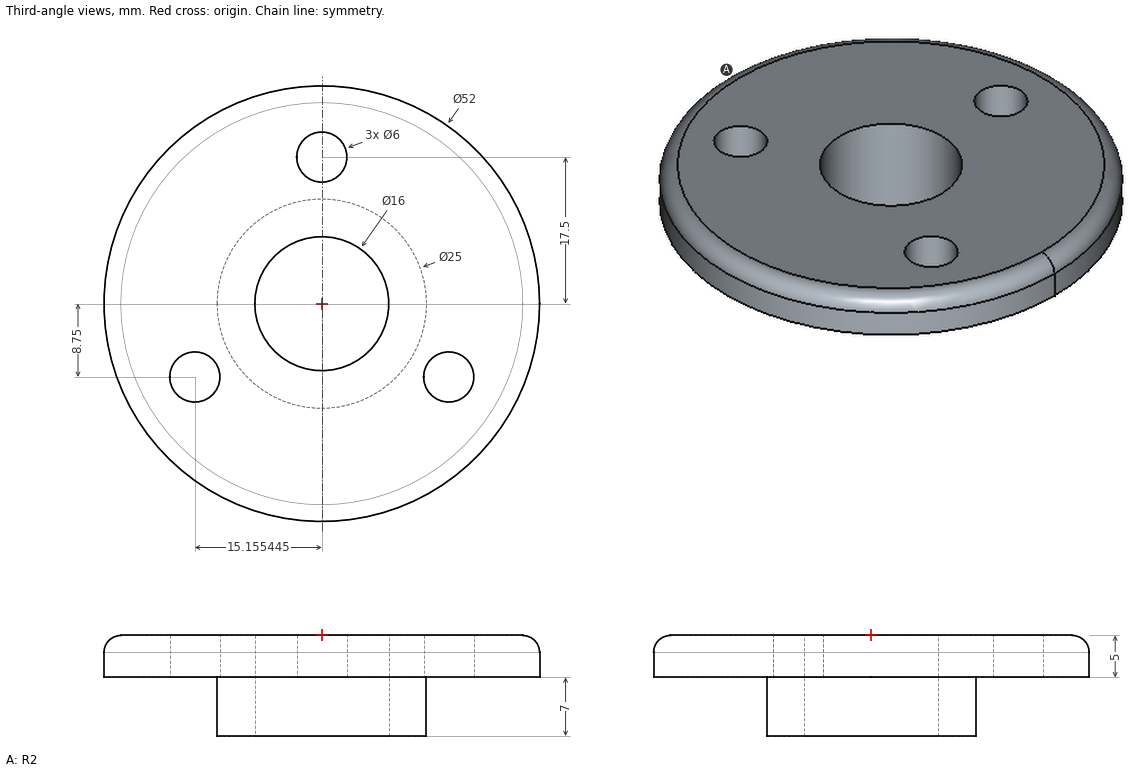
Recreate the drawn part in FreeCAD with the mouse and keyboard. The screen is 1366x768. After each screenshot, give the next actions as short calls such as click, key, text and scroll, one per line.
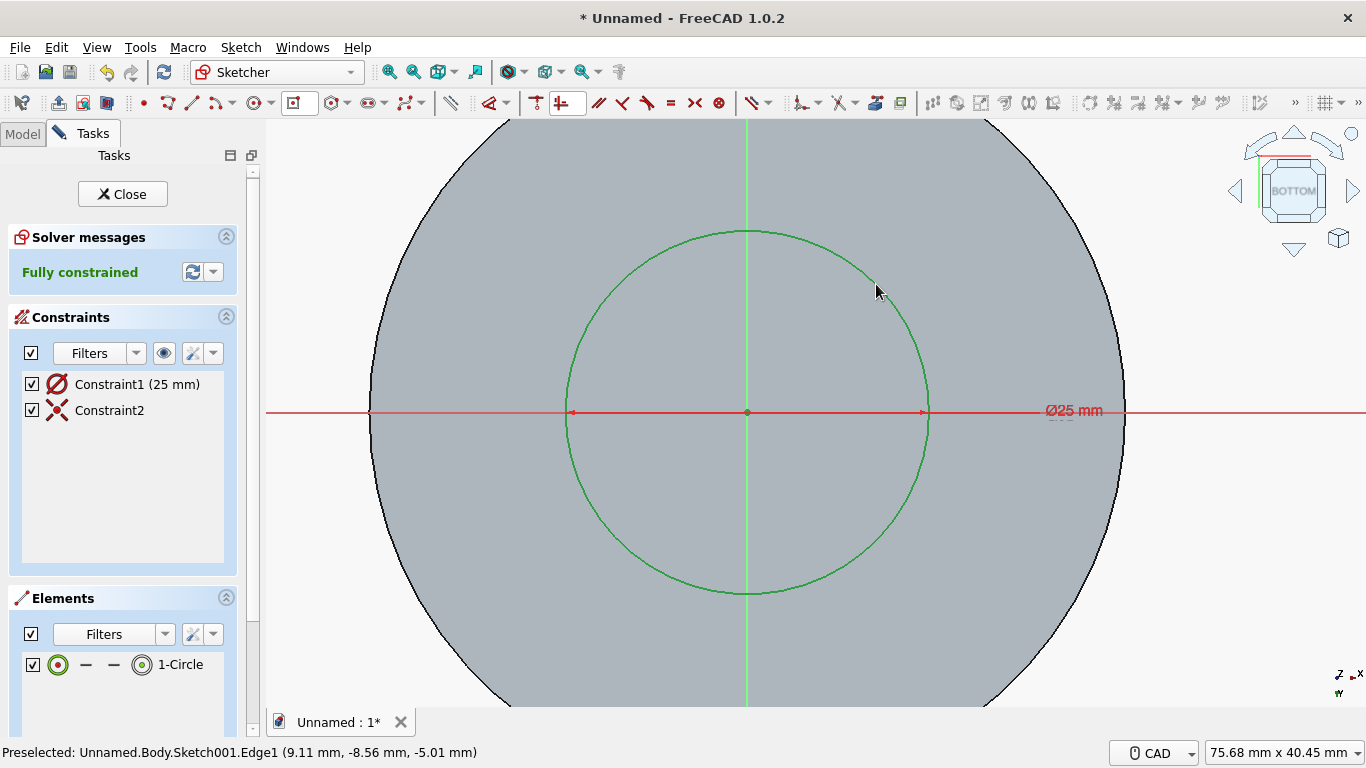
click(123, 194)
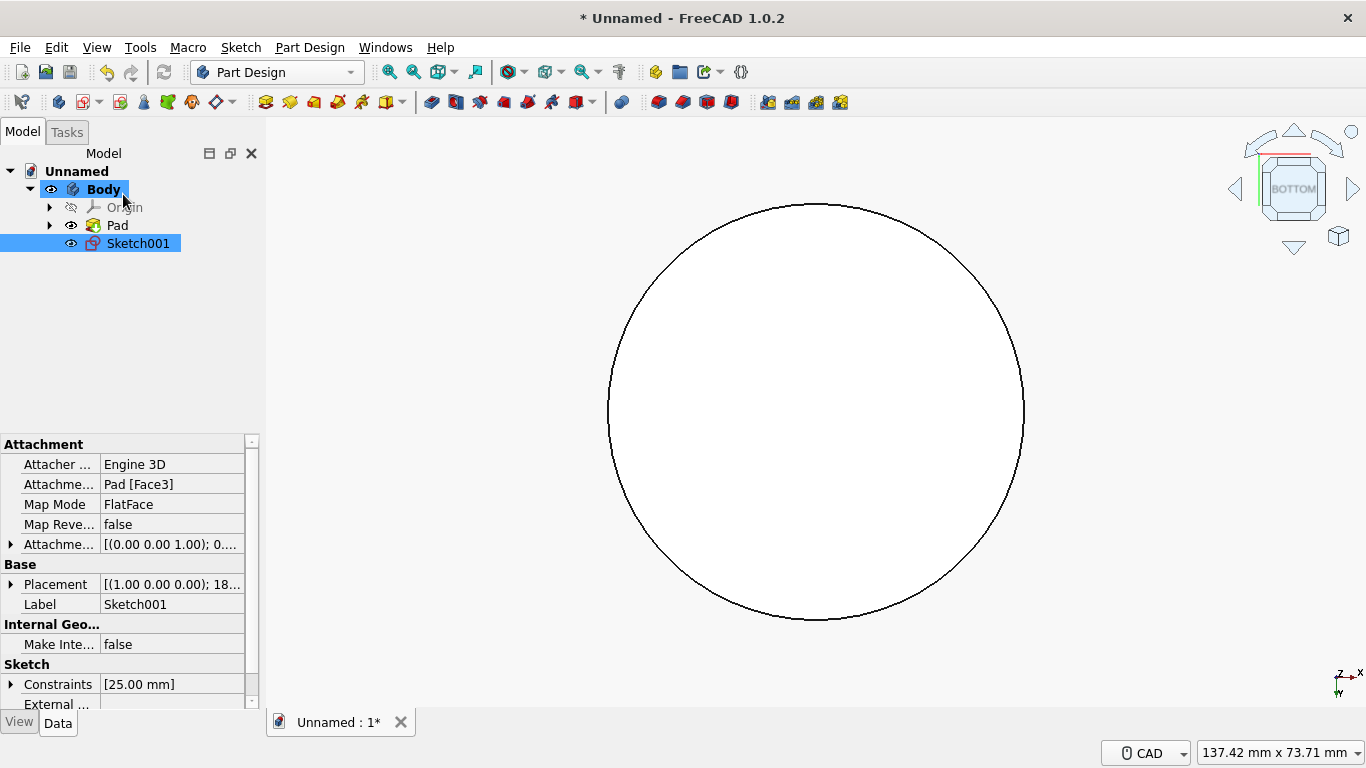
click(266, 102)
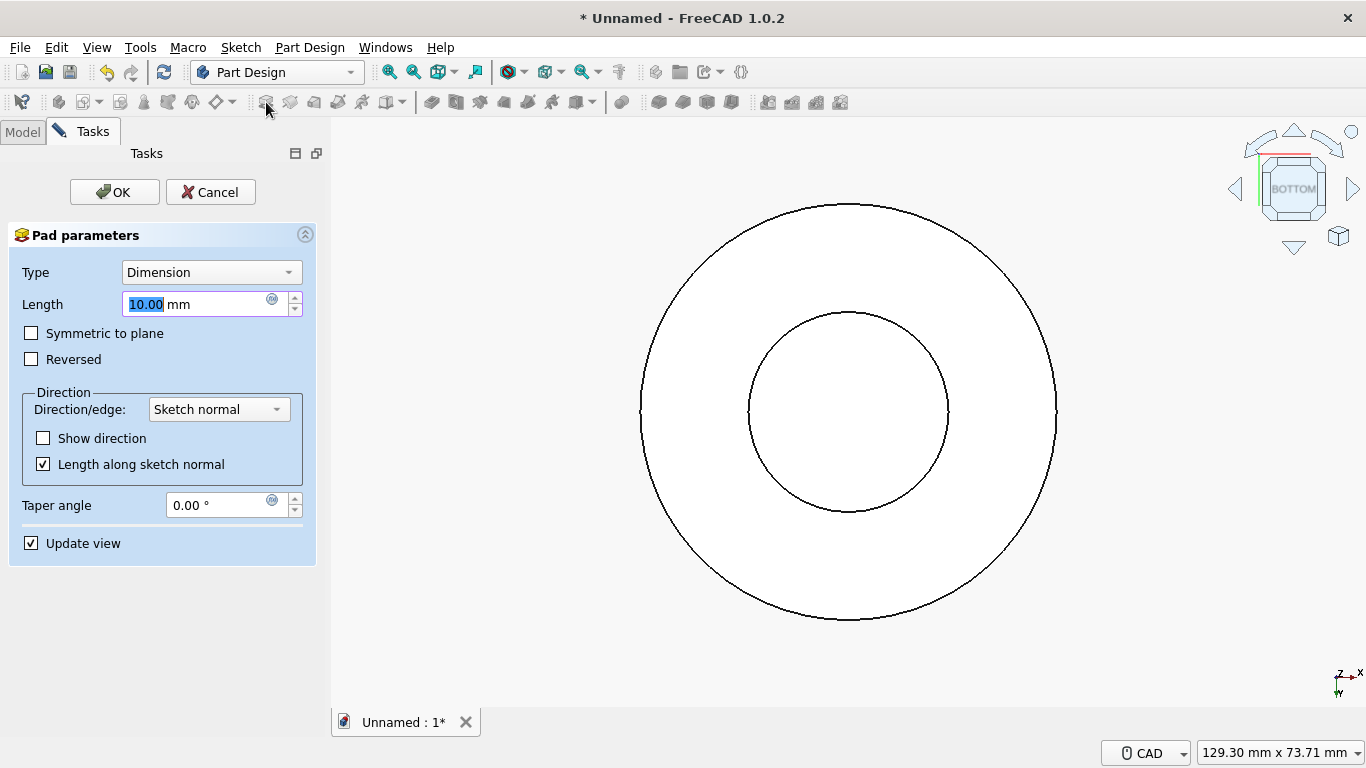
text(7)
key(Tab)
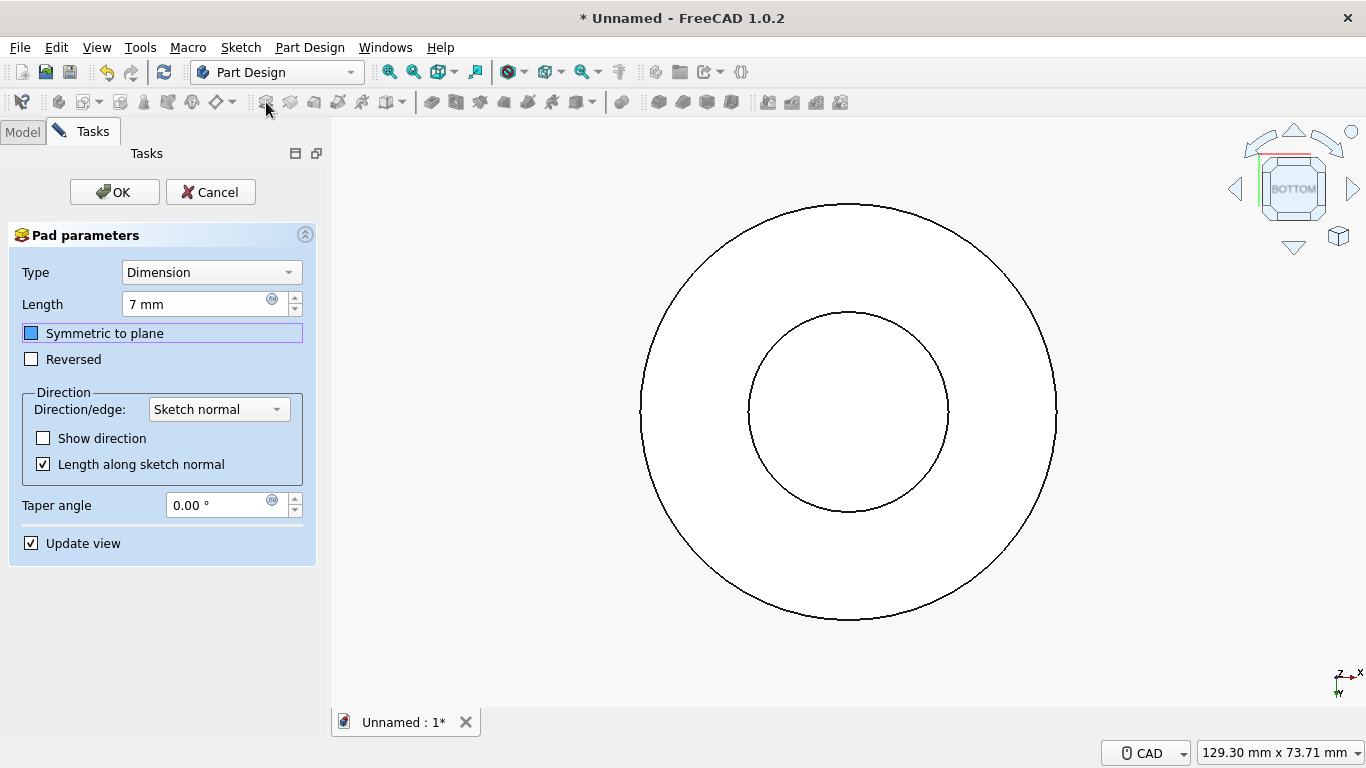
click(115, 192)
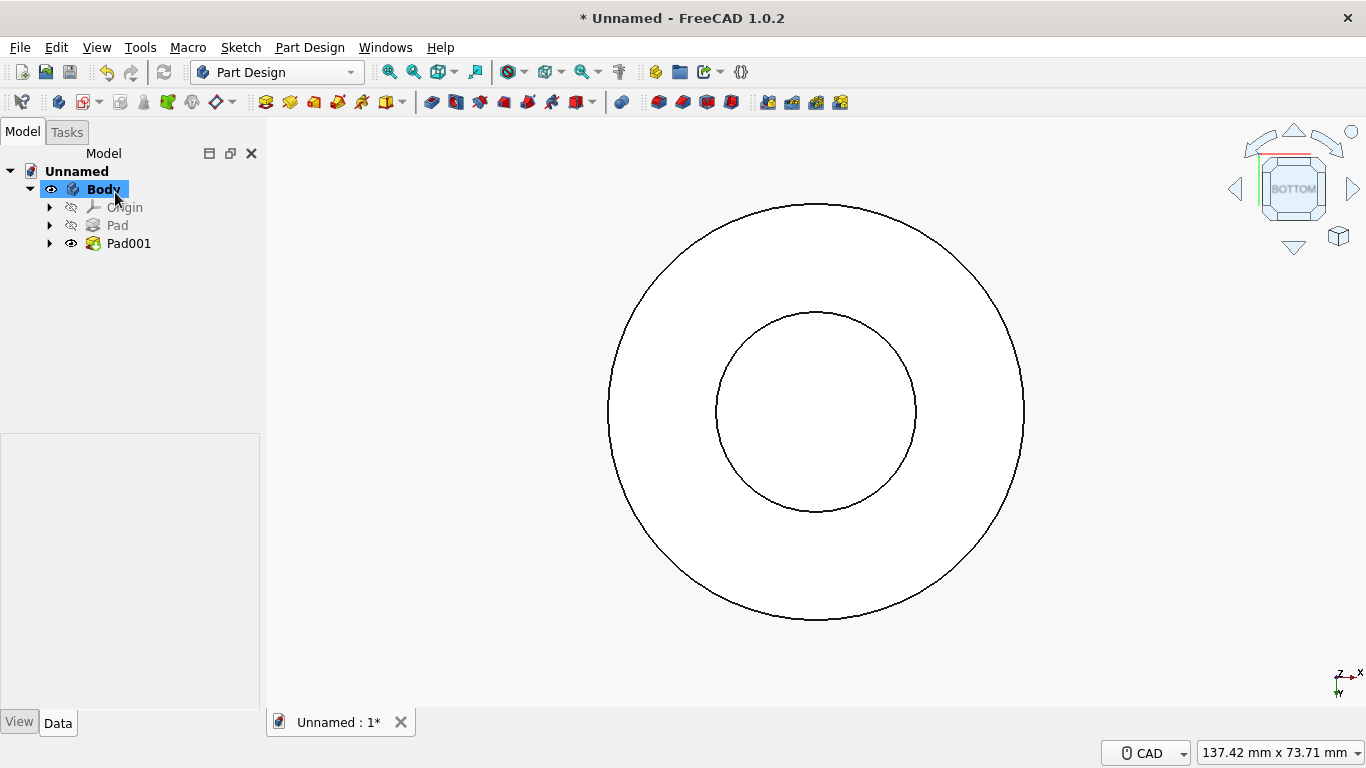
click(816, 411)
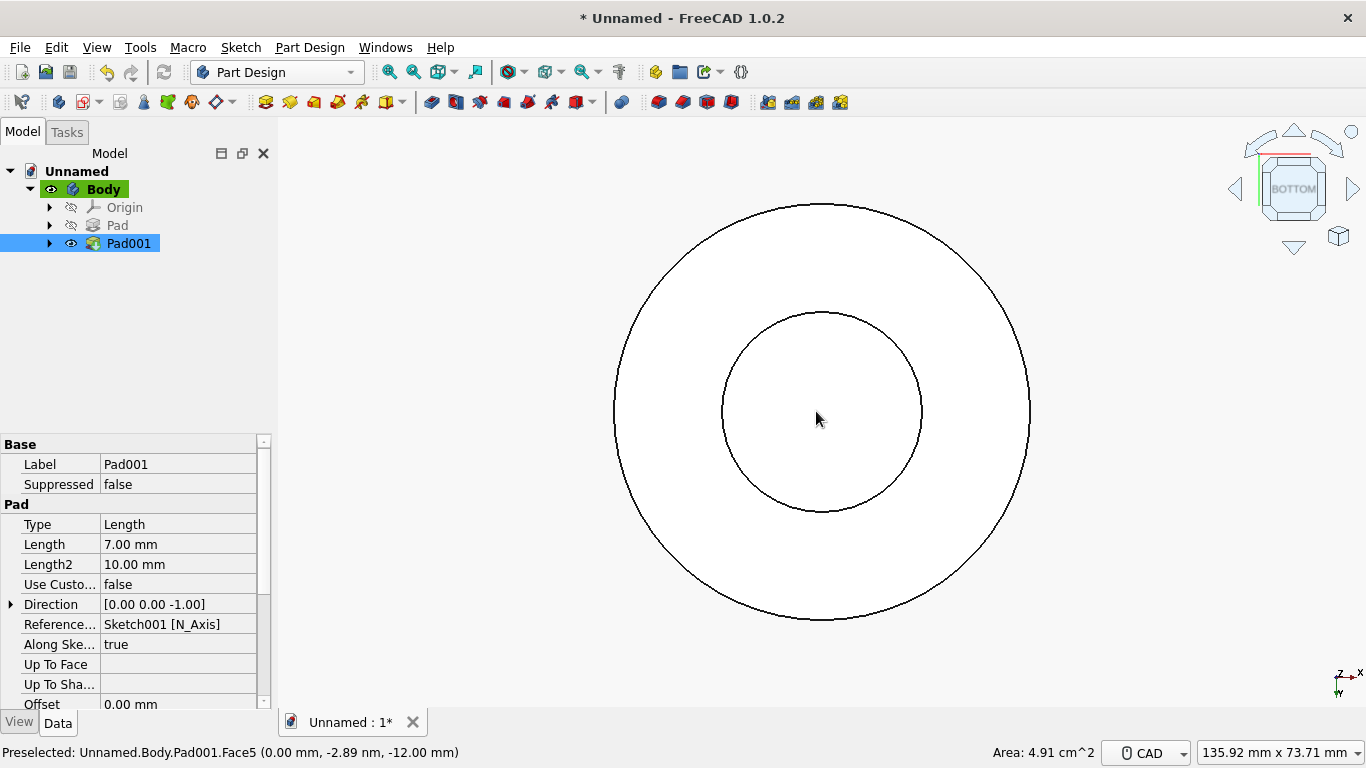
click(84, 102)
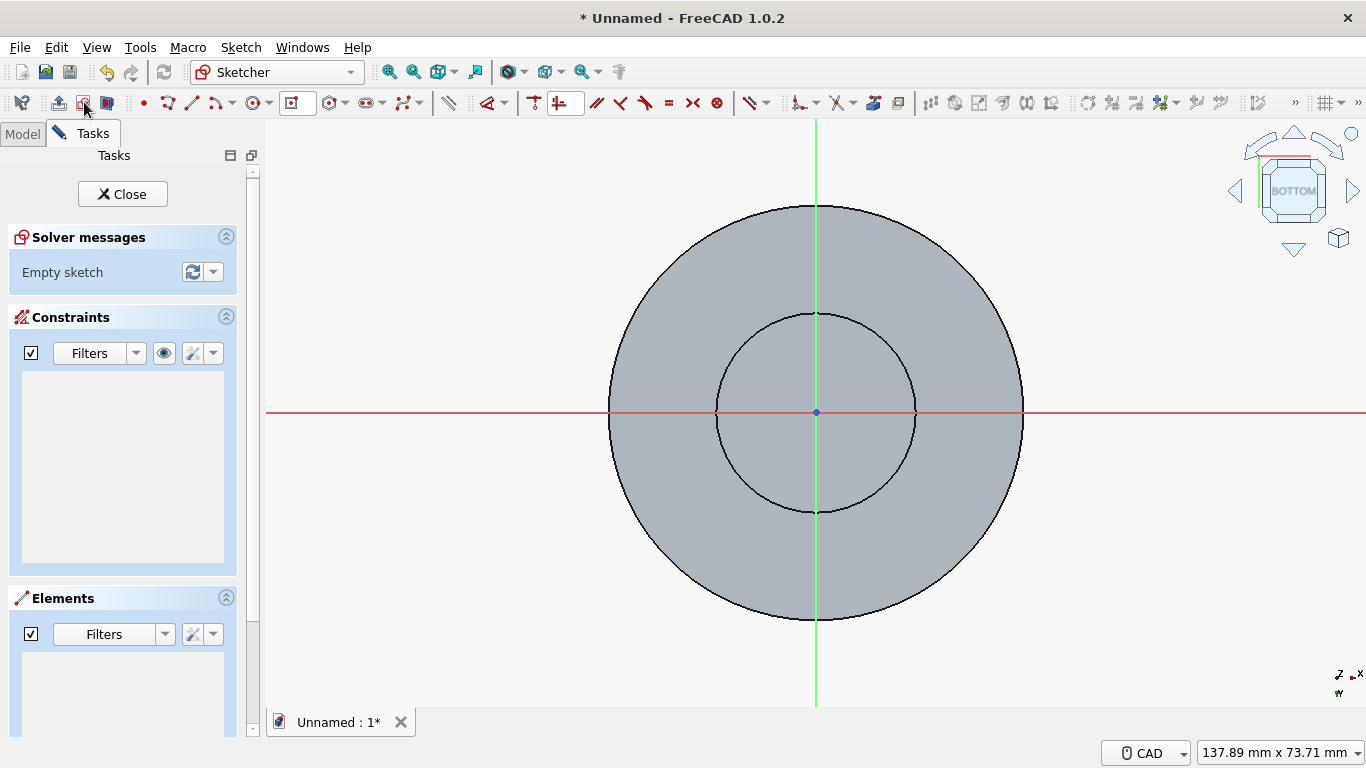
scroll(856, 413, up, 5)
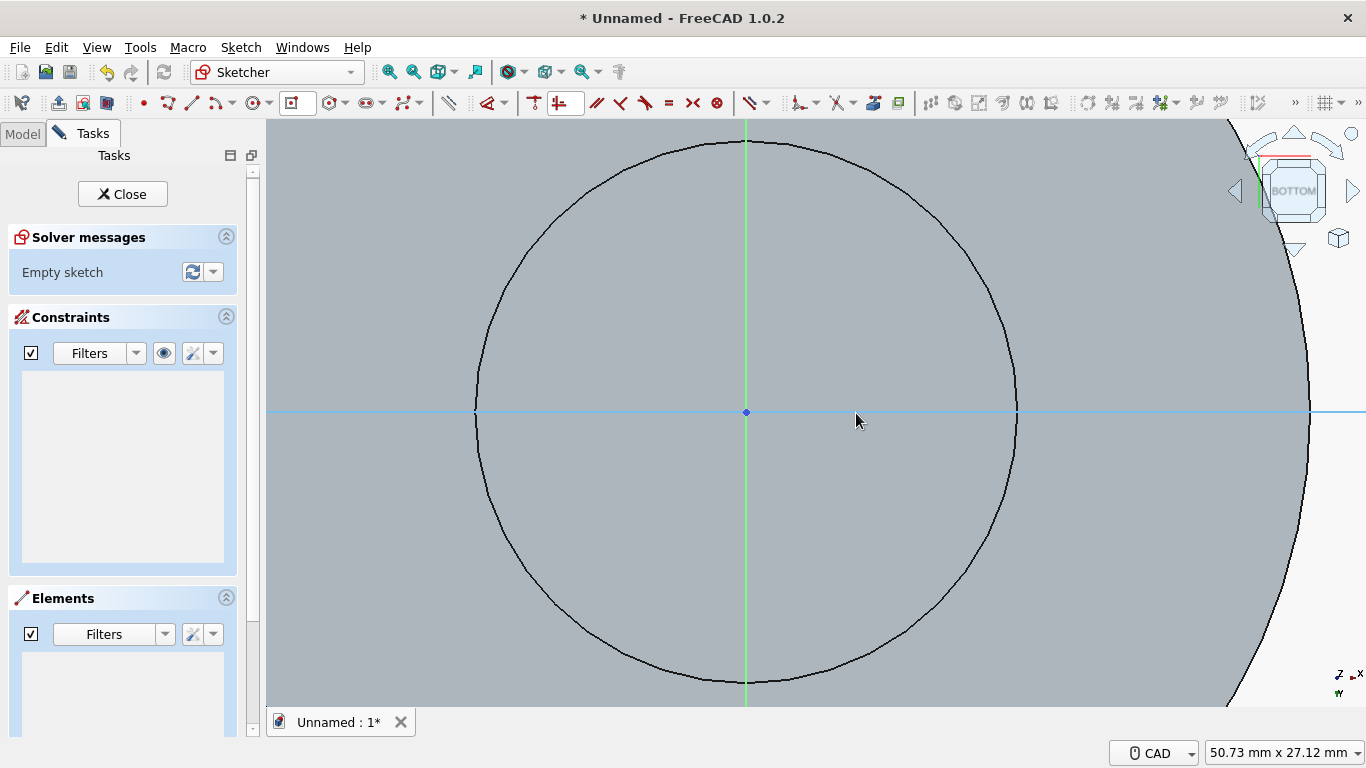
click(254, 104)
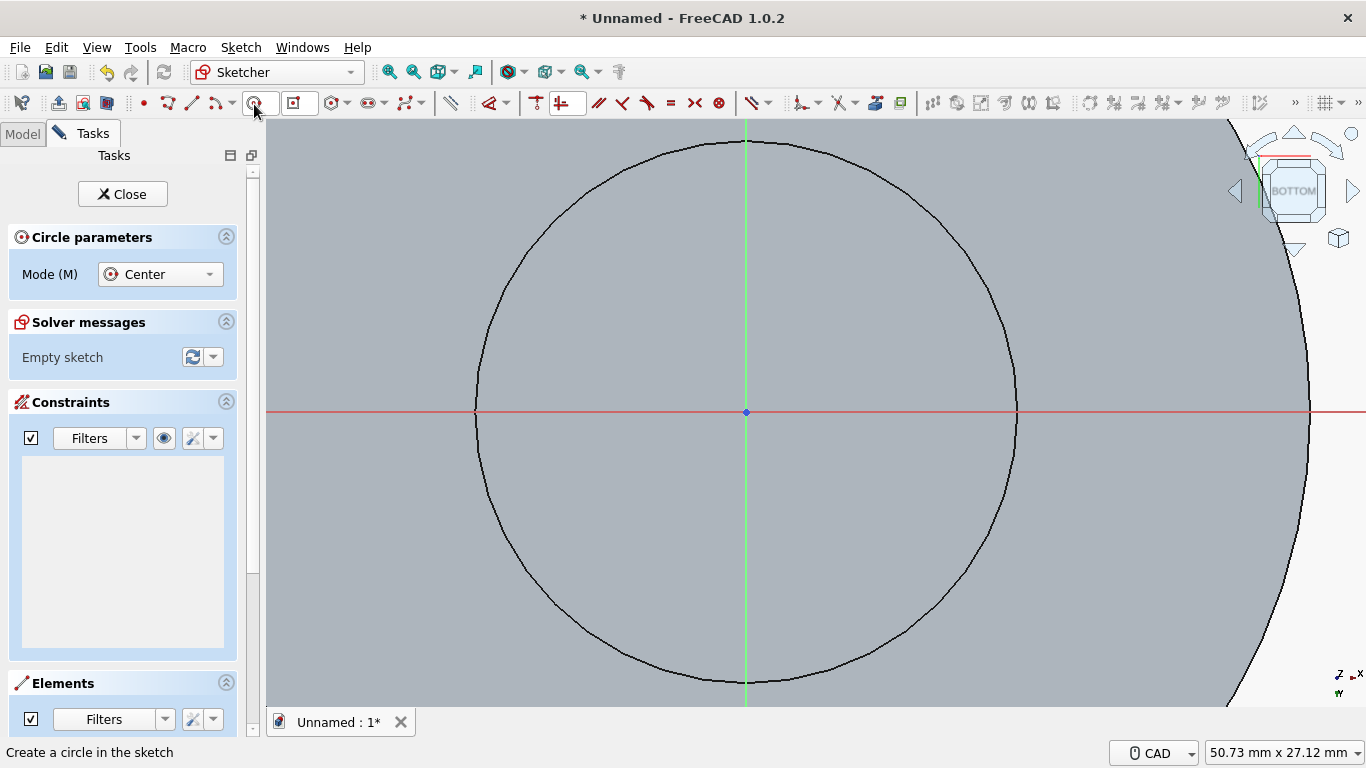
click(746, 412)
move(869, 289)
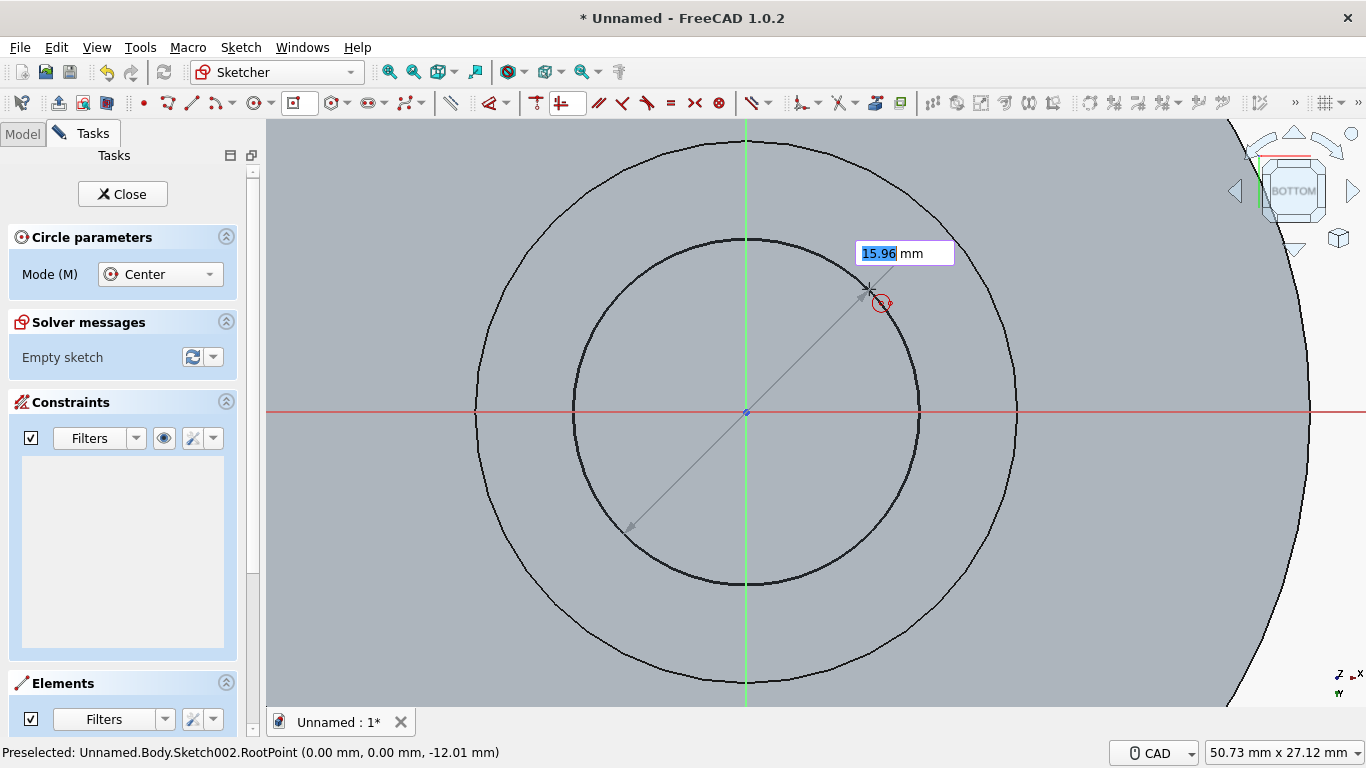
text(16)
key(Return)
key(Escape)